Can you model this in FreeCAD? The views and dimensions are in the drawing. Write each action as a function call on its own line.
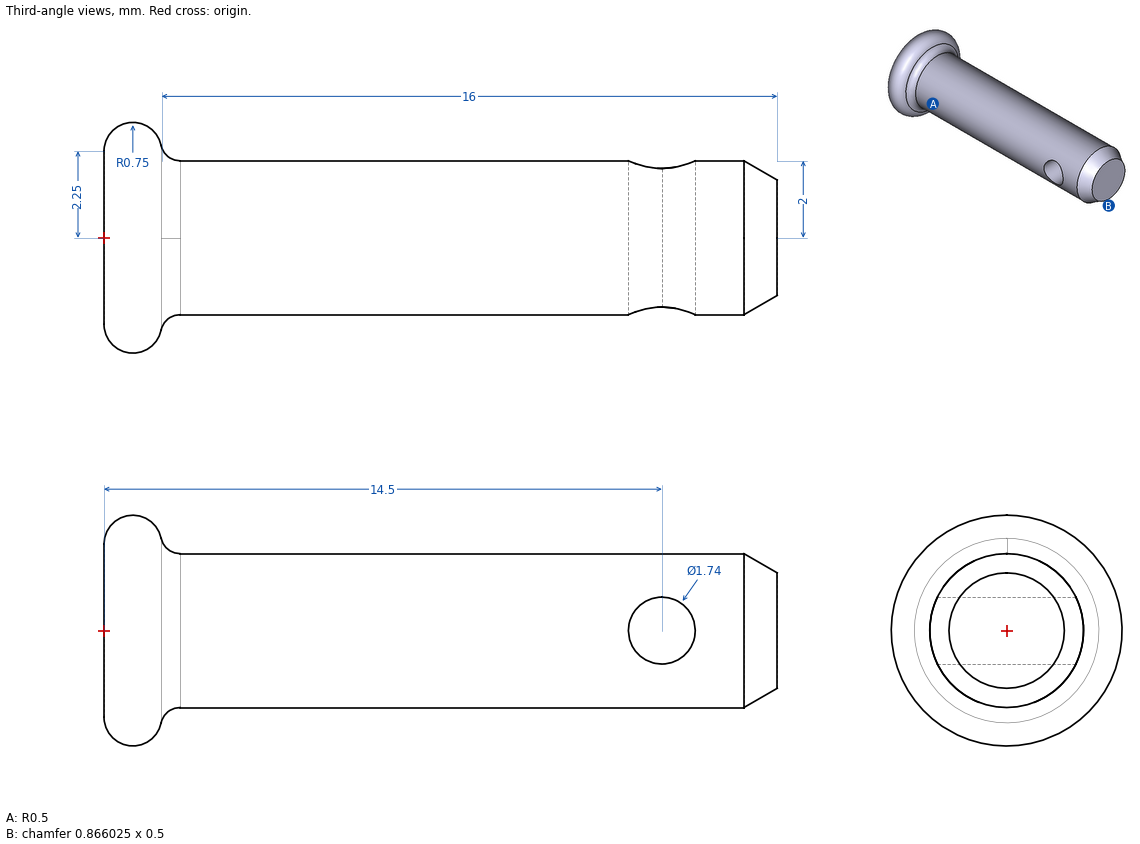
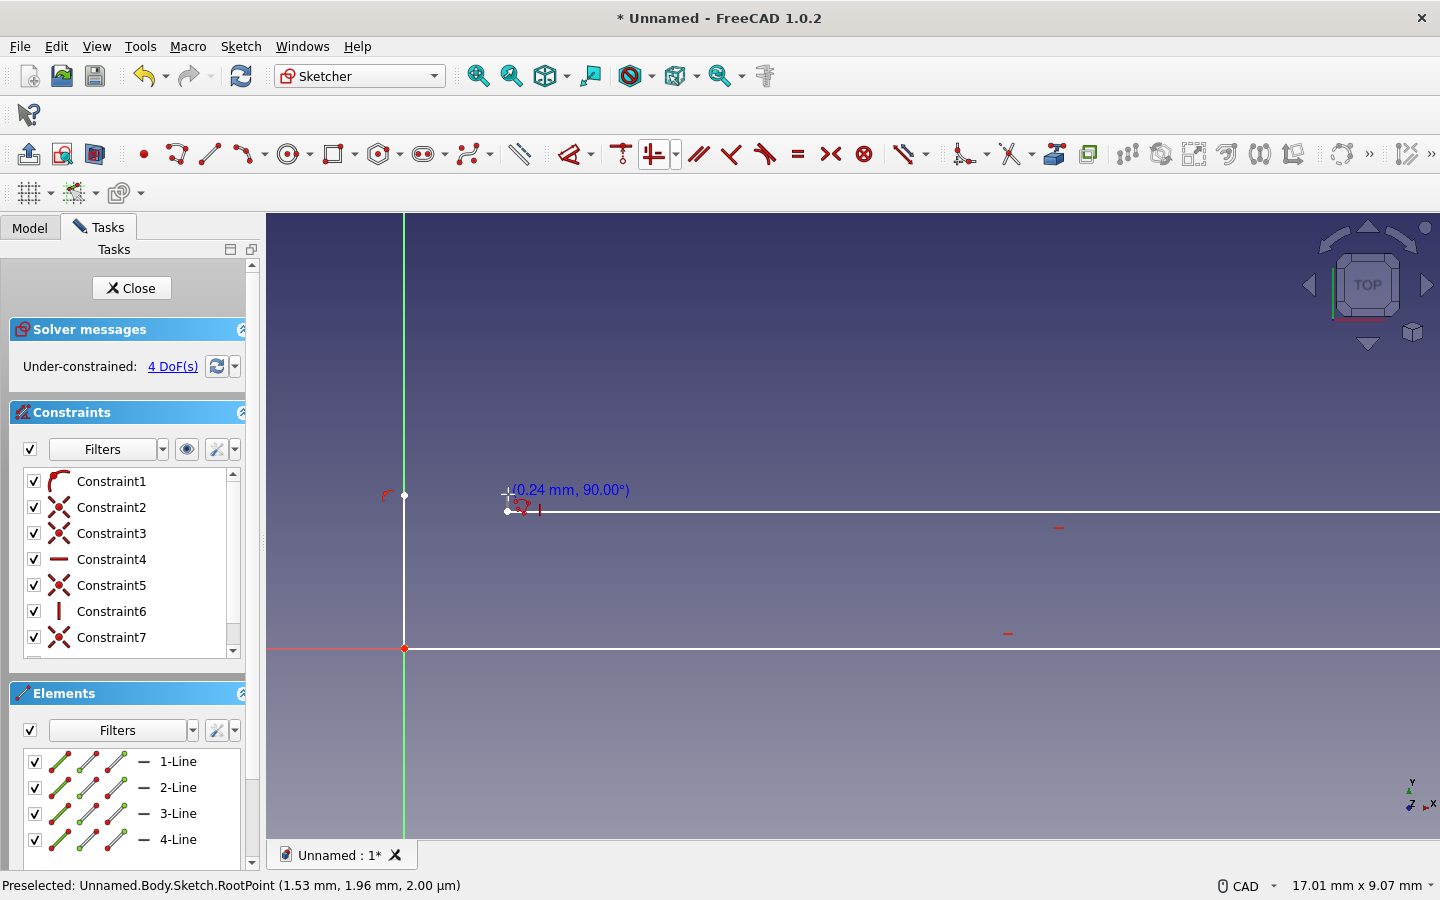
click(508, 493)
right_click(508, 493)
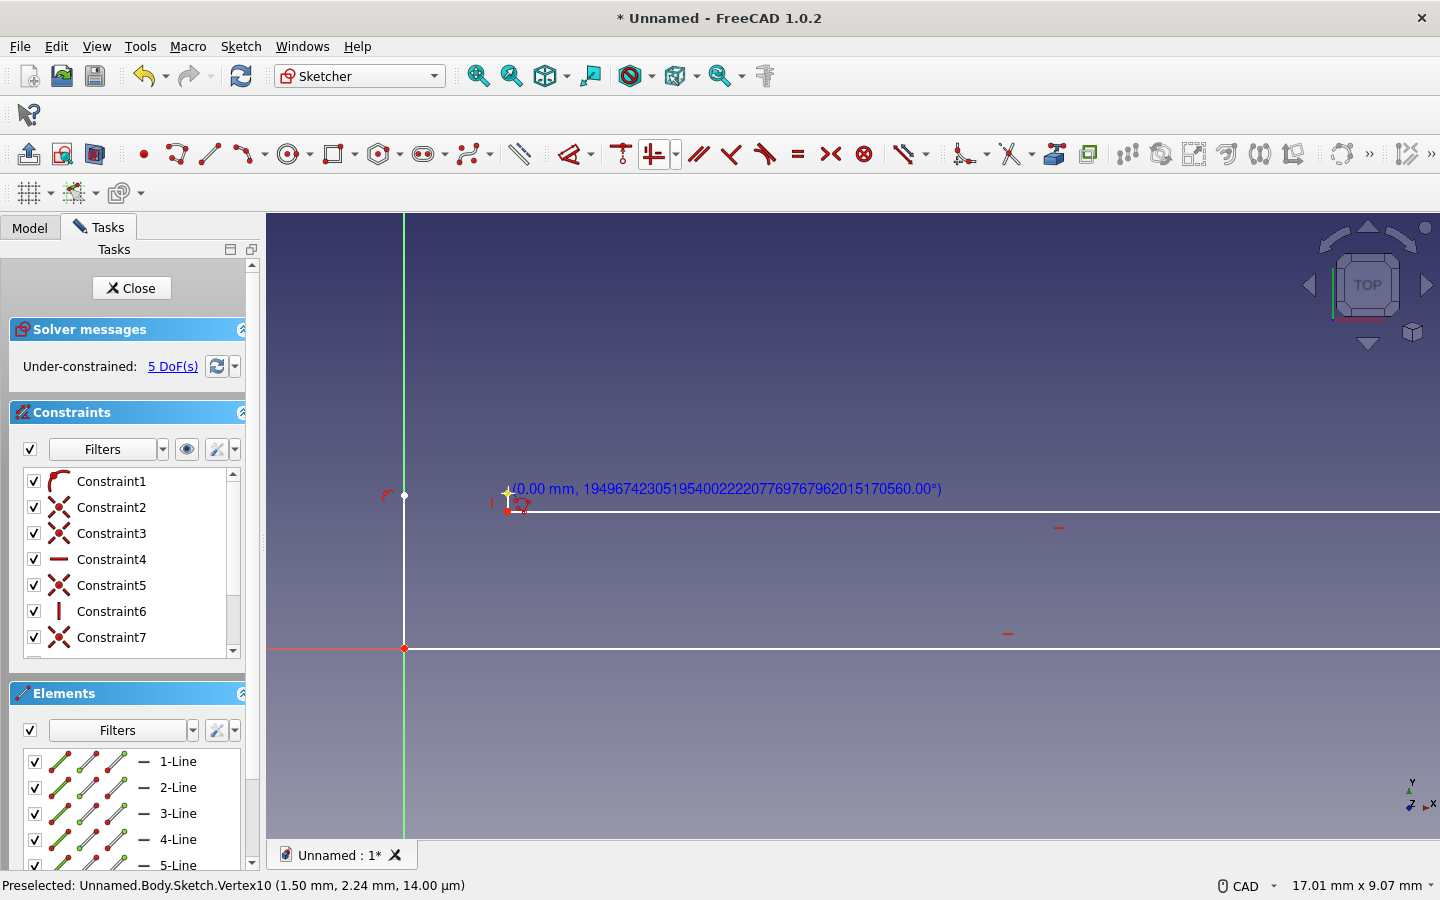
click(242, 154)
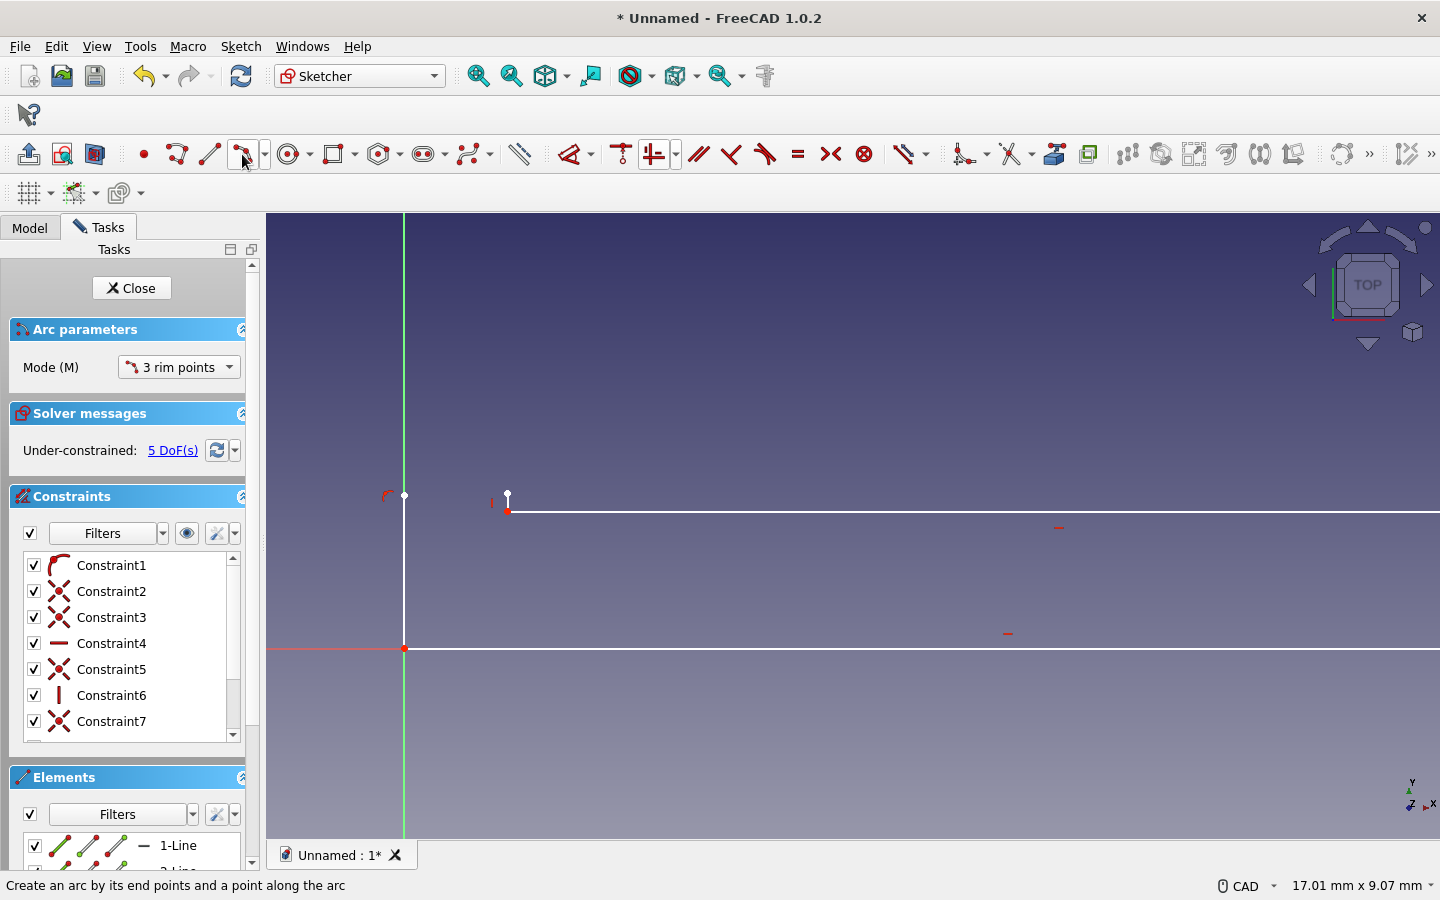
scroll(508, 493, up, 4)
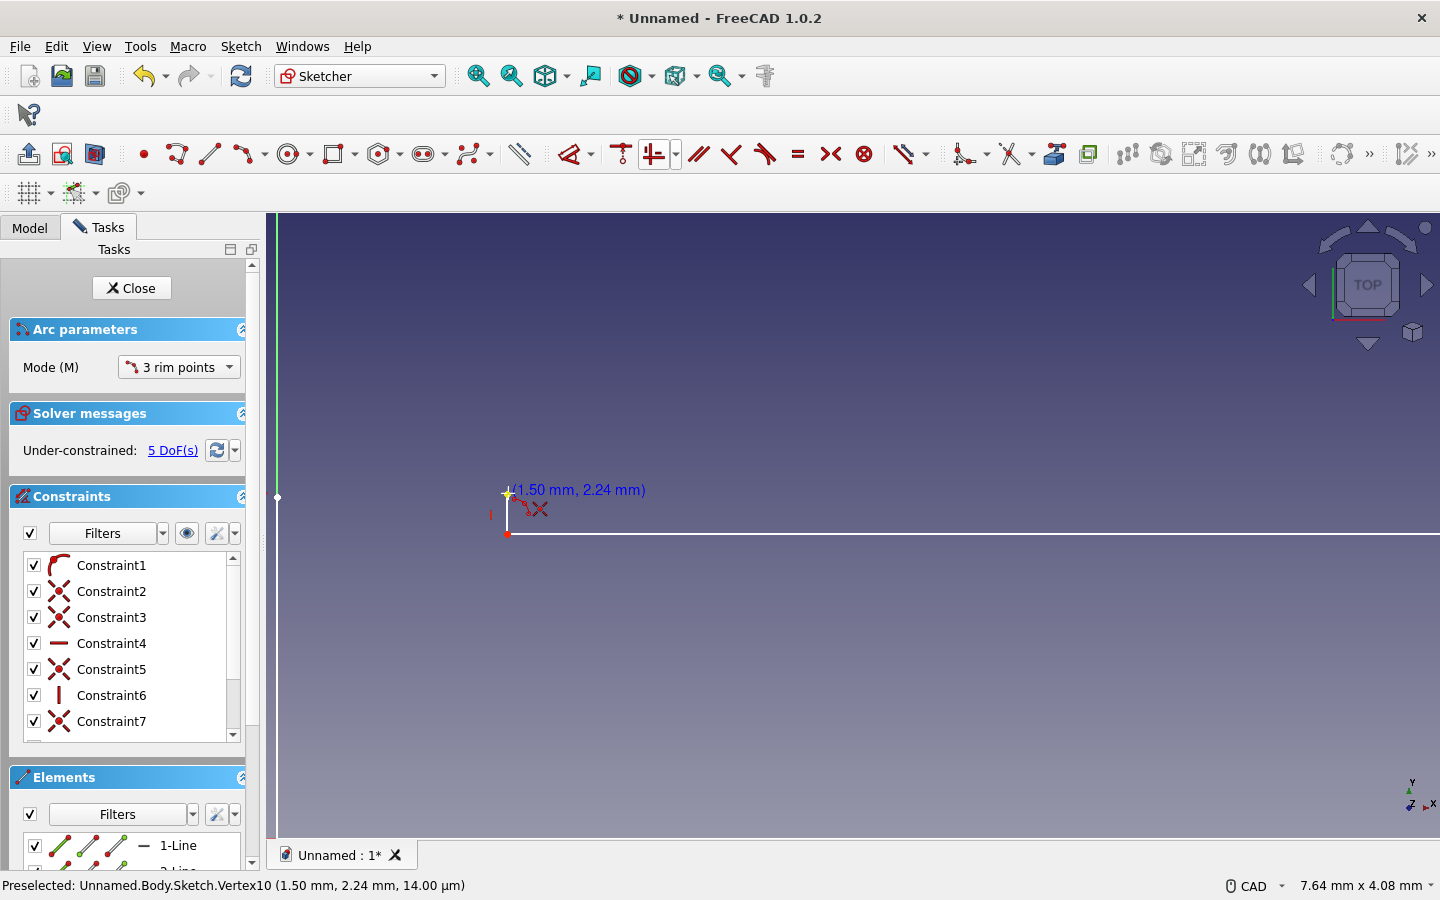
click(507, 495)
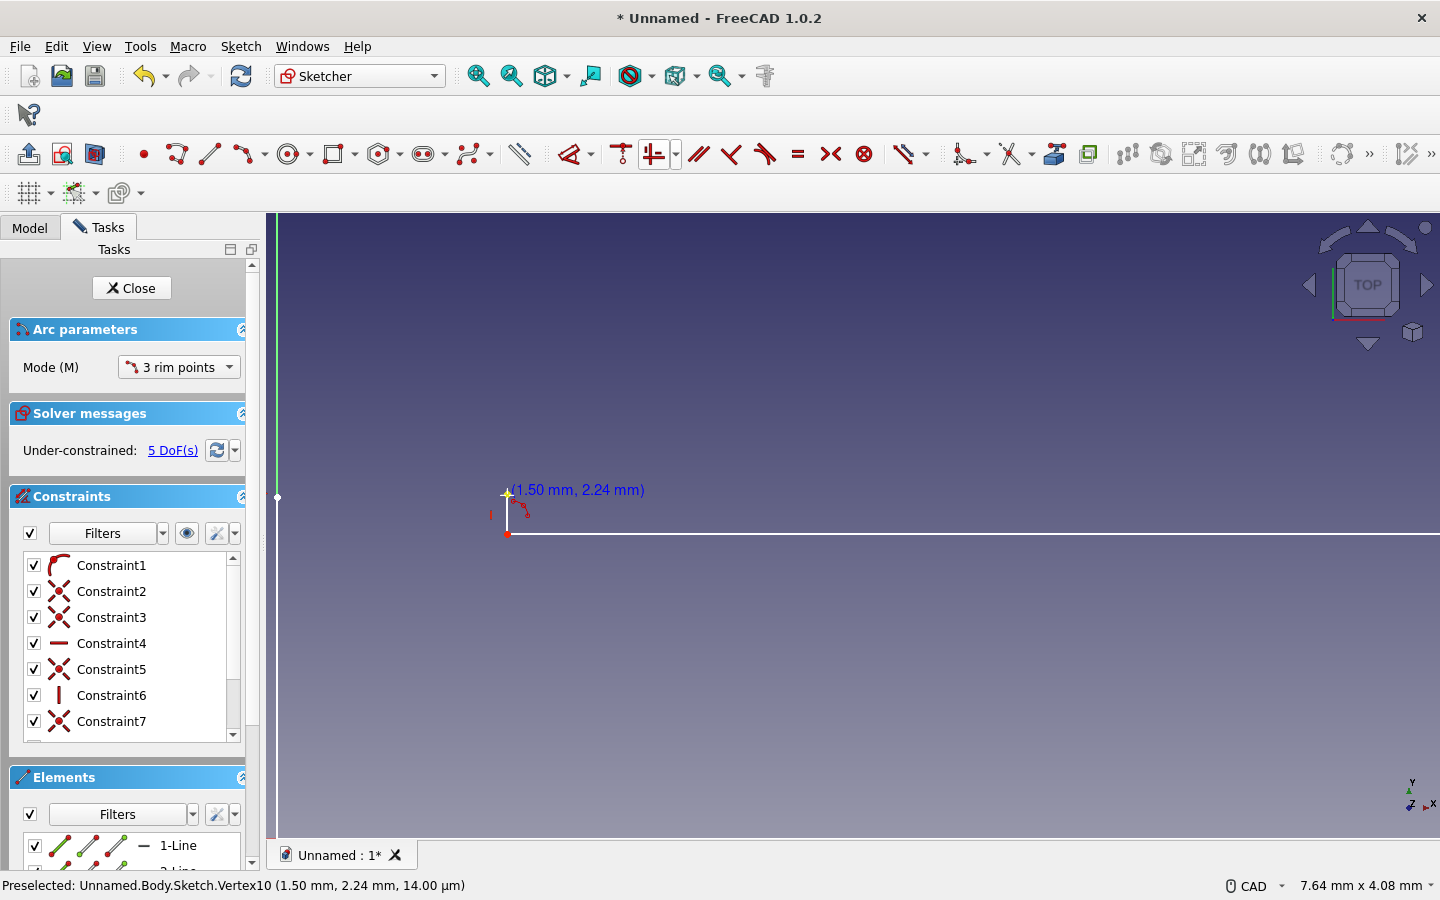
scroll(511, 499, down, 7)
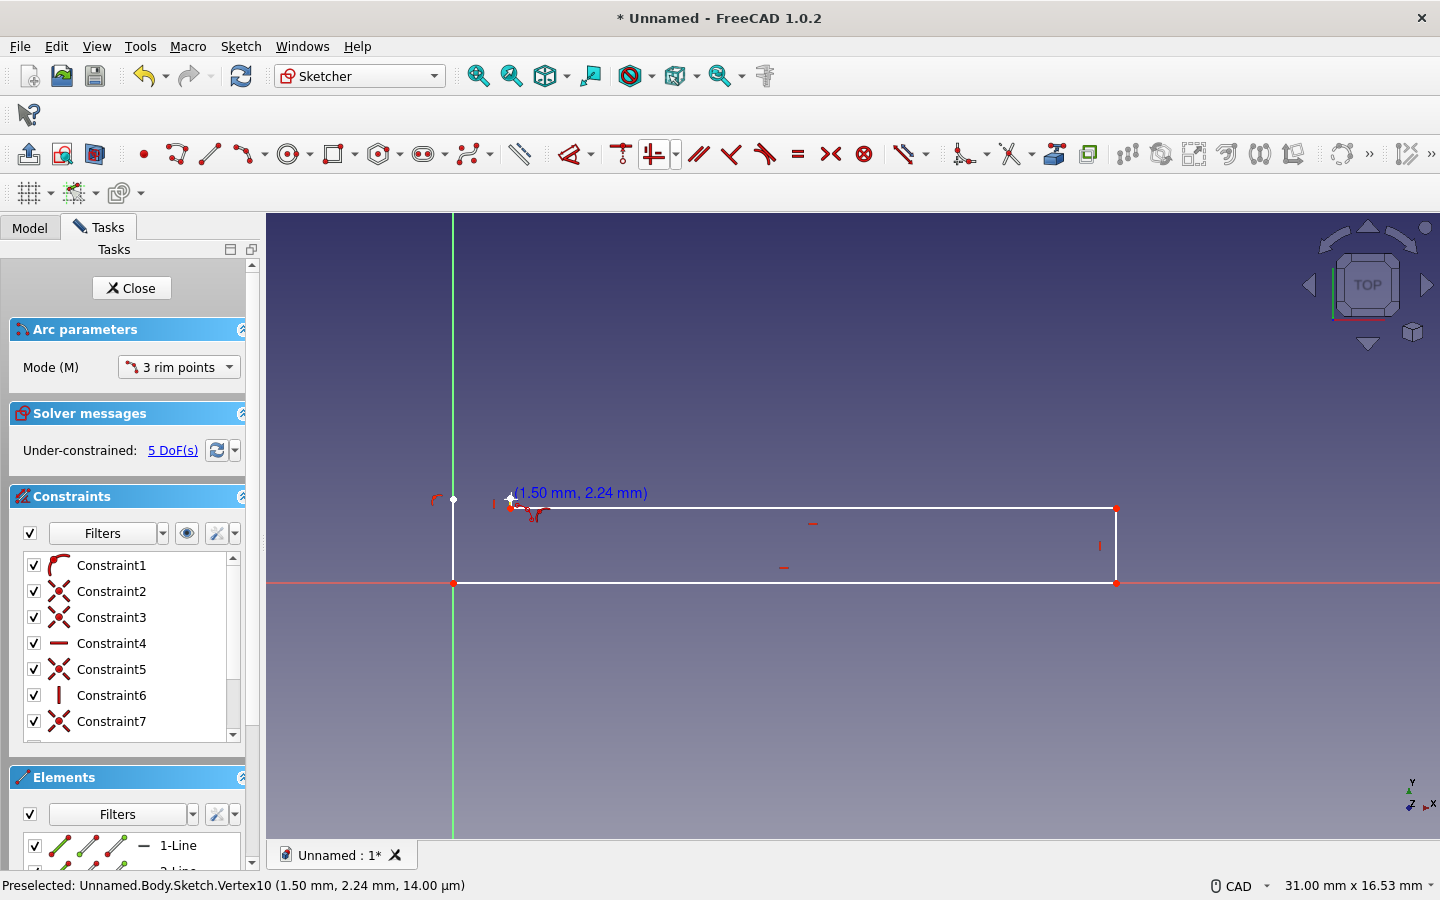
click(453, 499)
click(482, 470)
key(Escape)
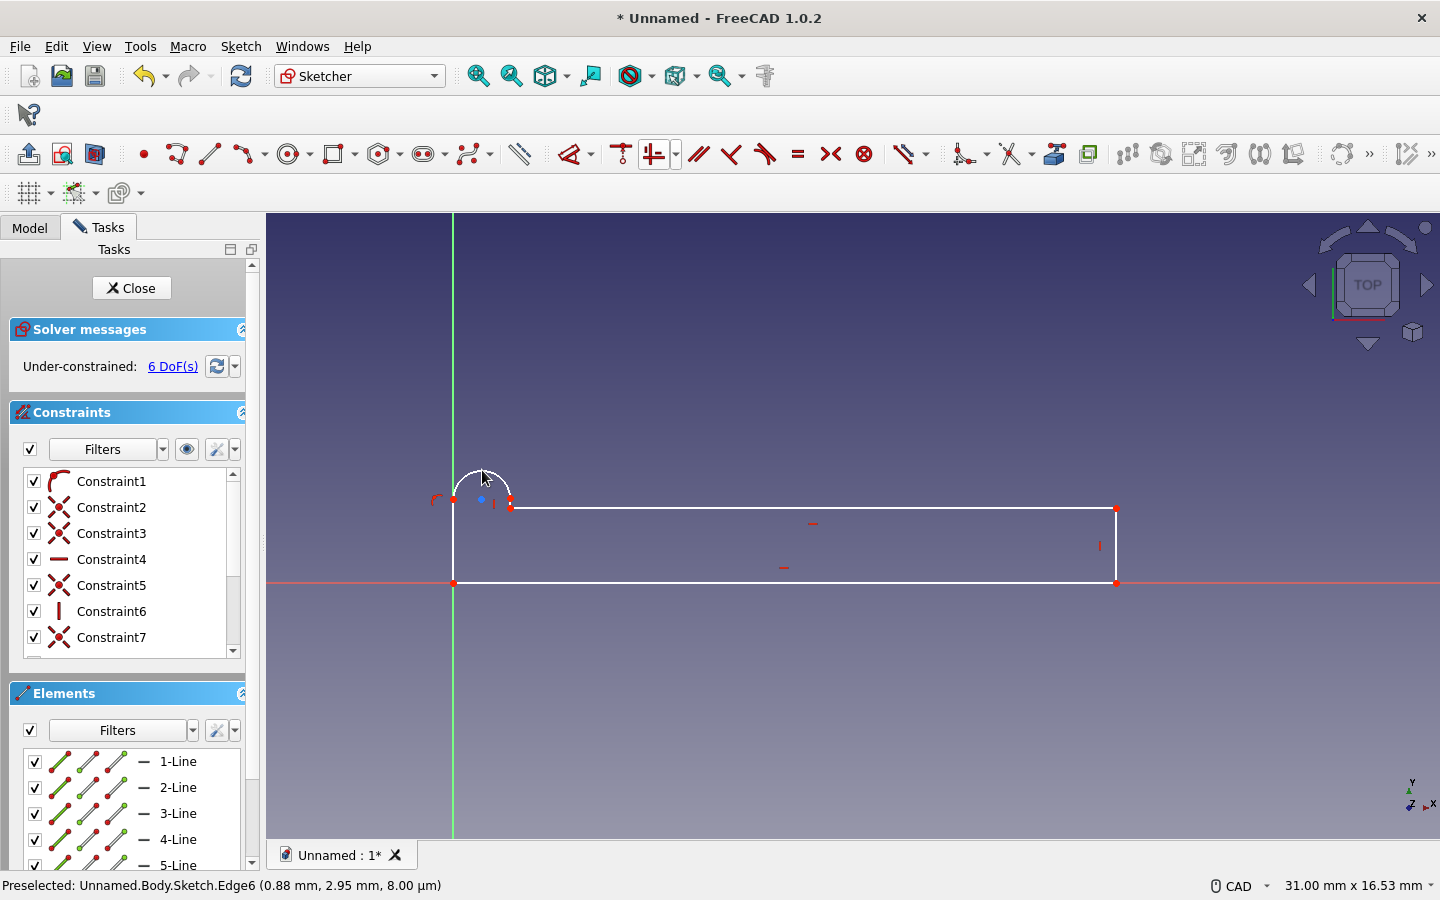
click(453, 524)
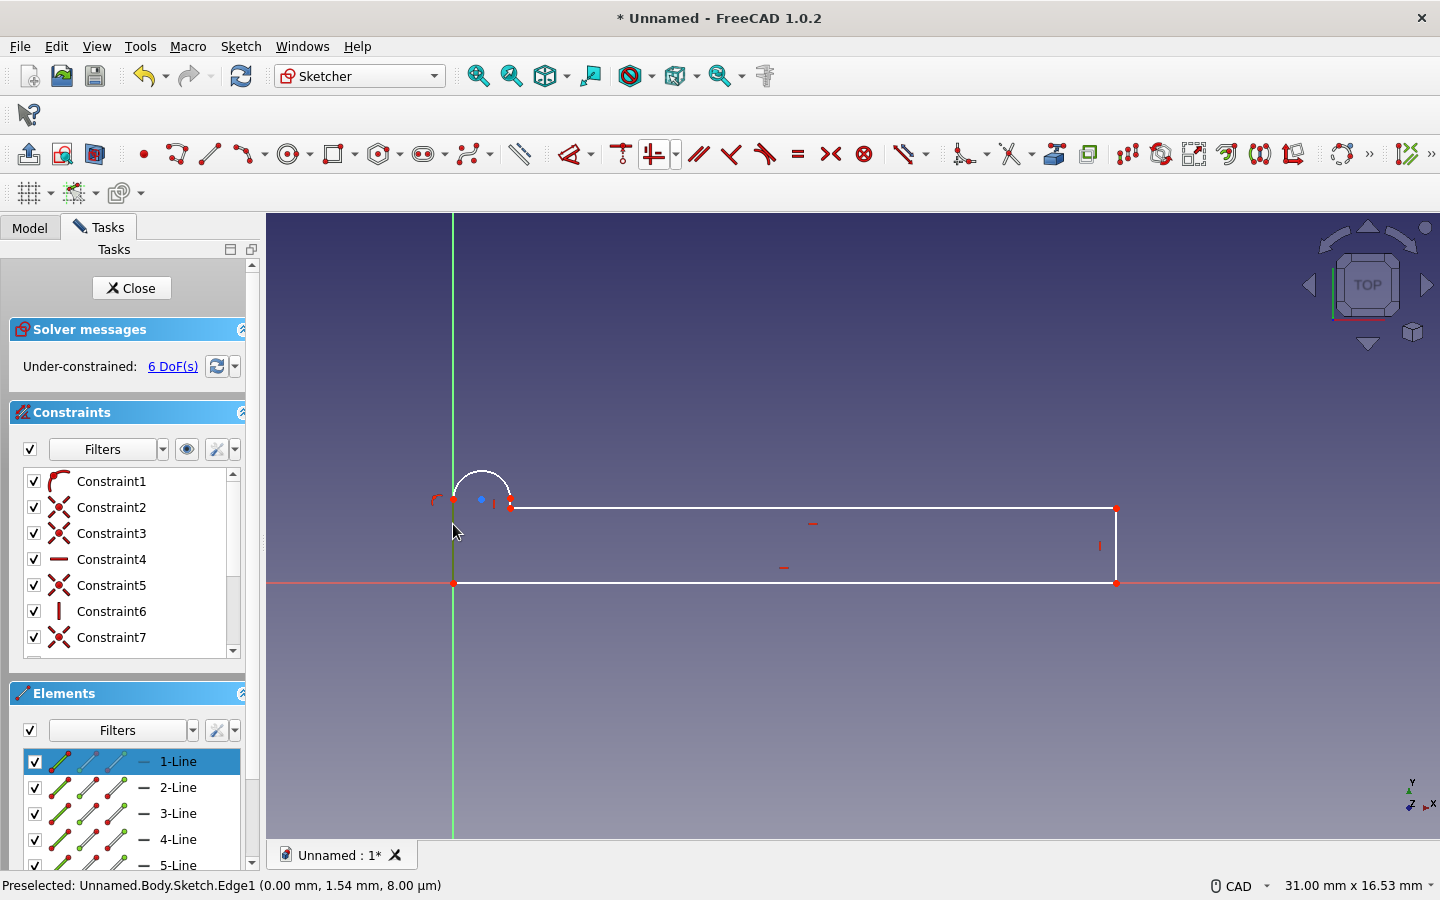
click(498, 476)